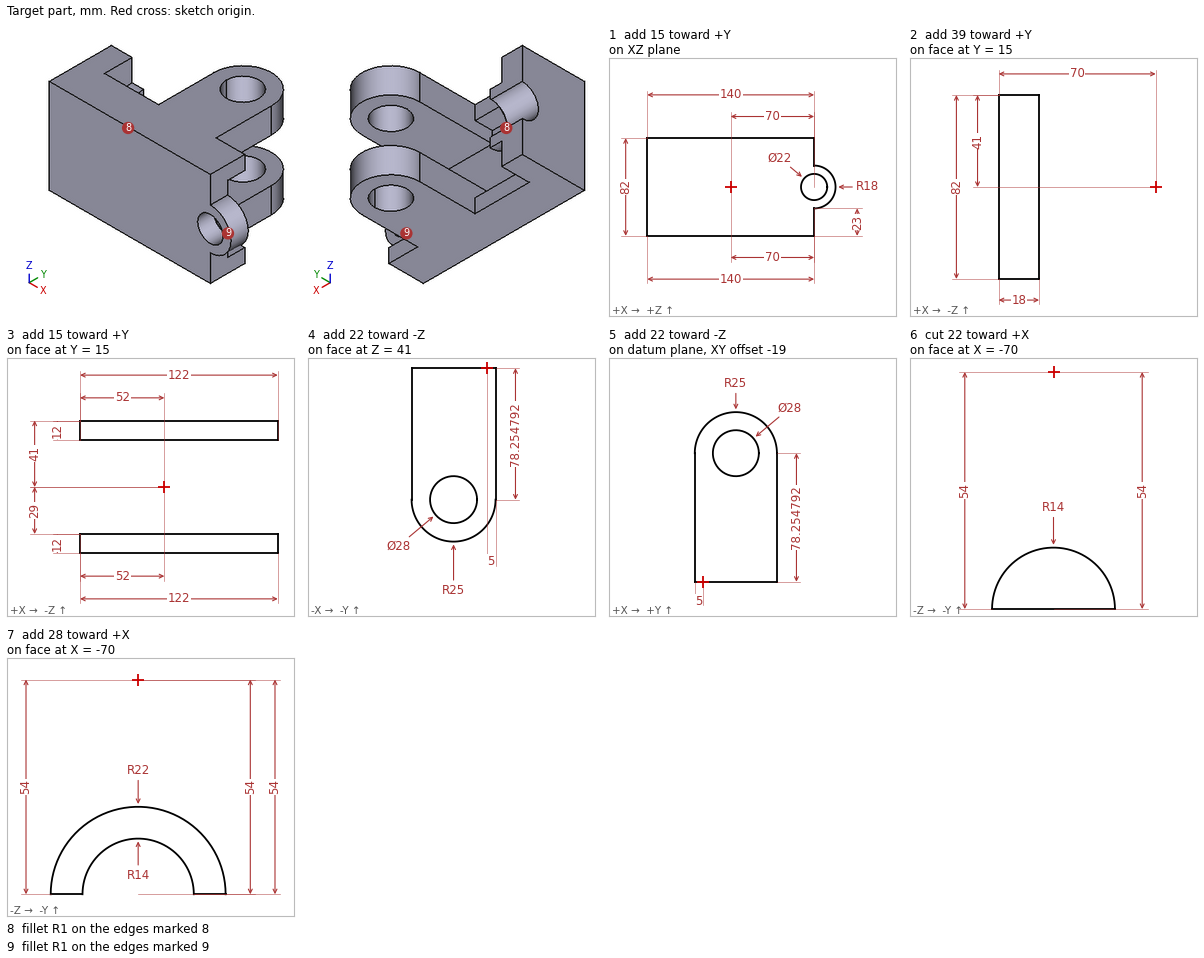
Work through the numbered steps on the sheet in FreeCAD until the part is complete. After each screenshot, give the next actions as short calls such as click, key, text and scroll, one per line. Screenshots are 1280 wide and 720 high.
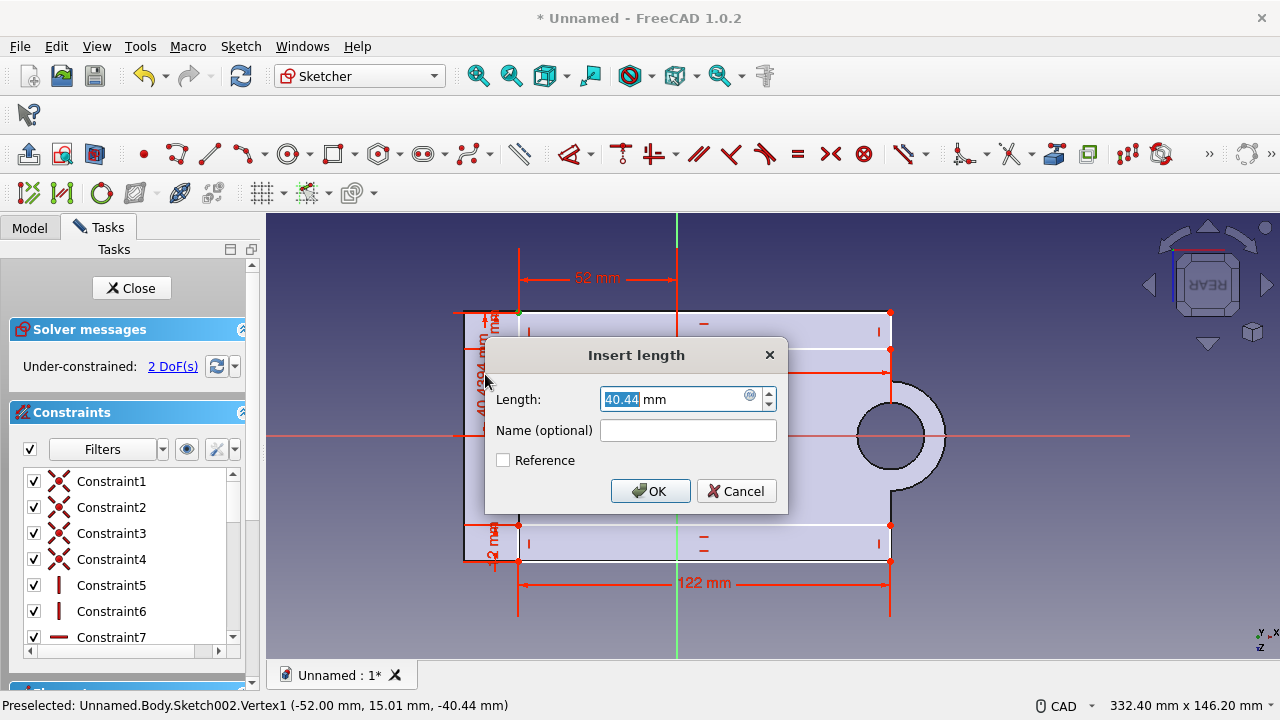
text(41)
key(Return)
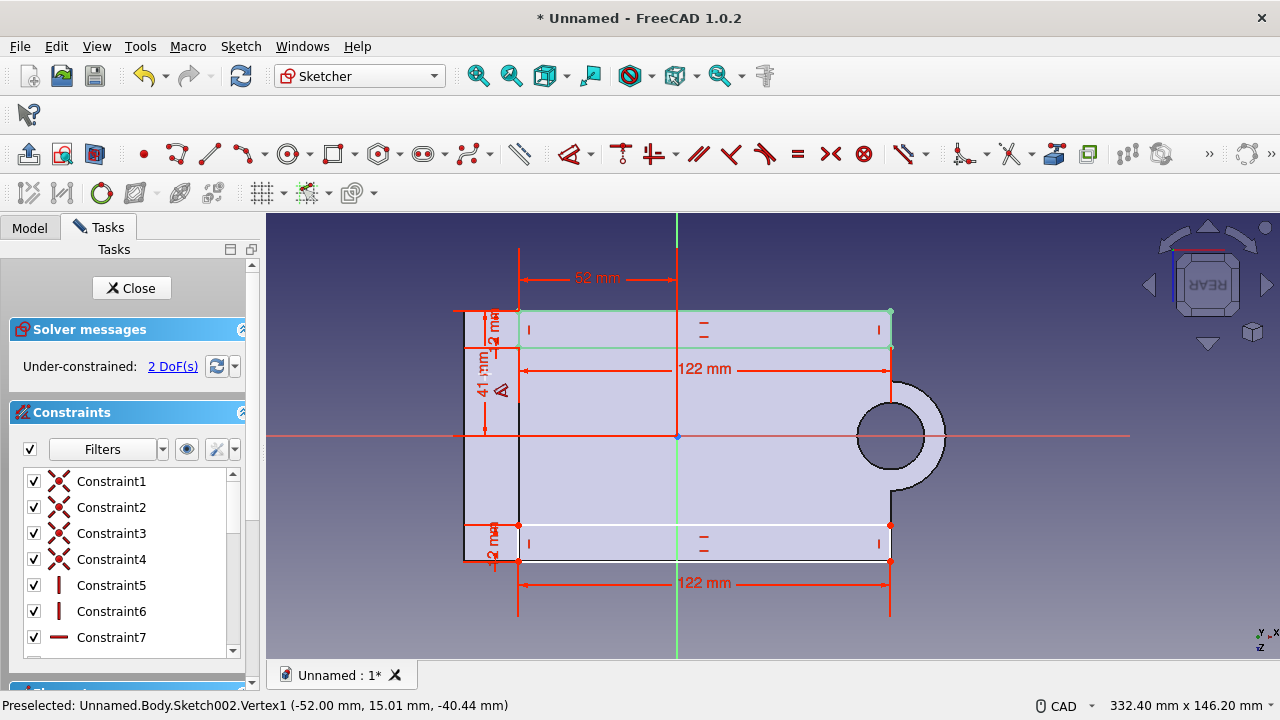
click(518, 525)
click(598, 402)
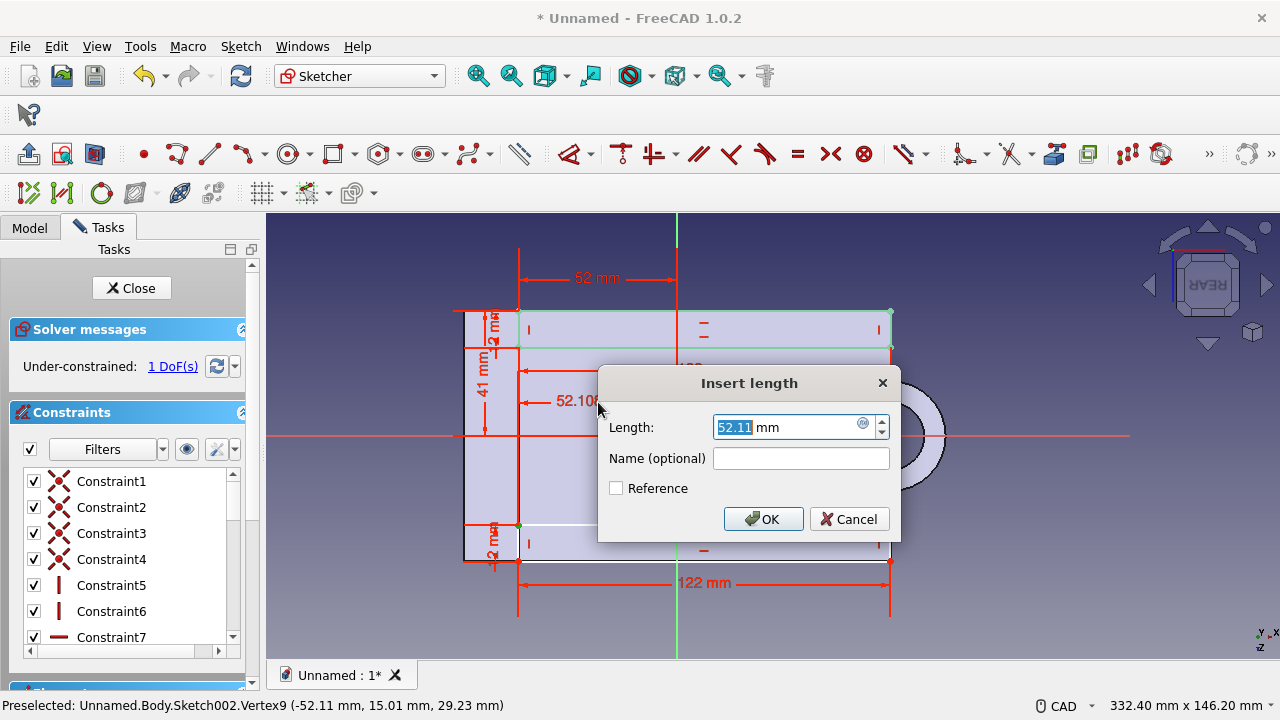
text(52)
key(Return)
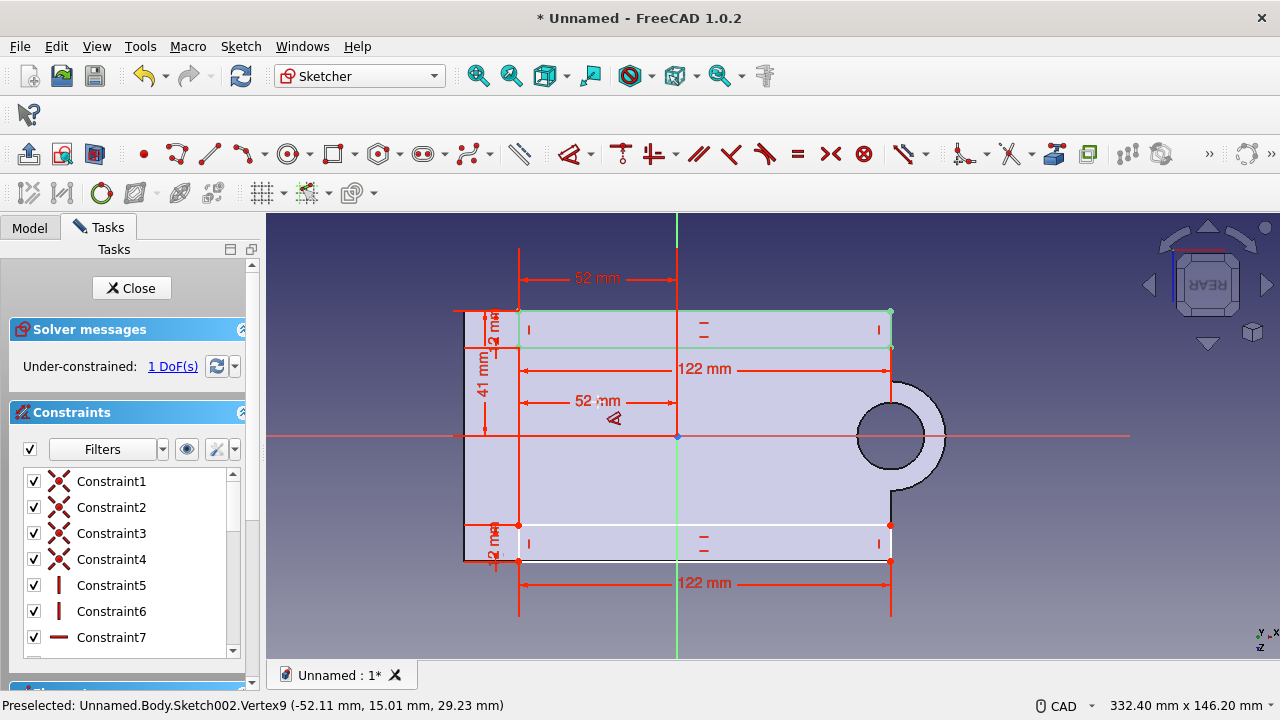
click(519, 525)
click(485, 481)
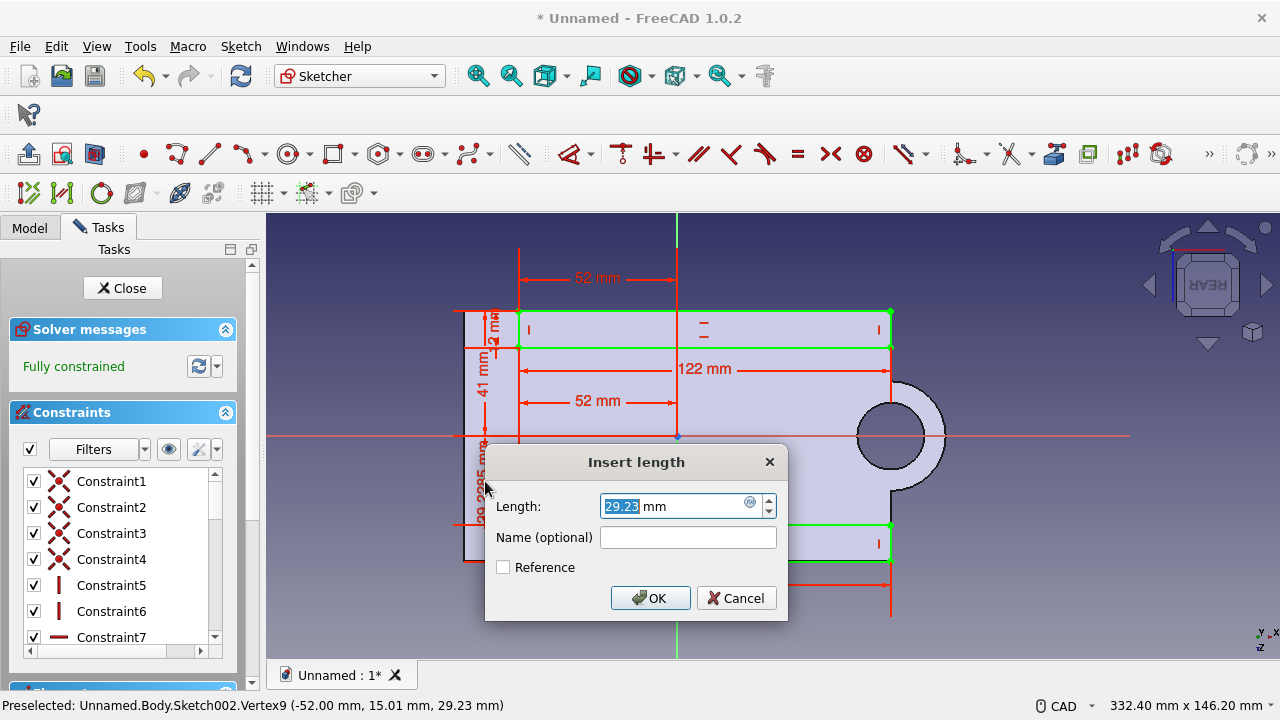
text(29)
key(Return)
key(Escape)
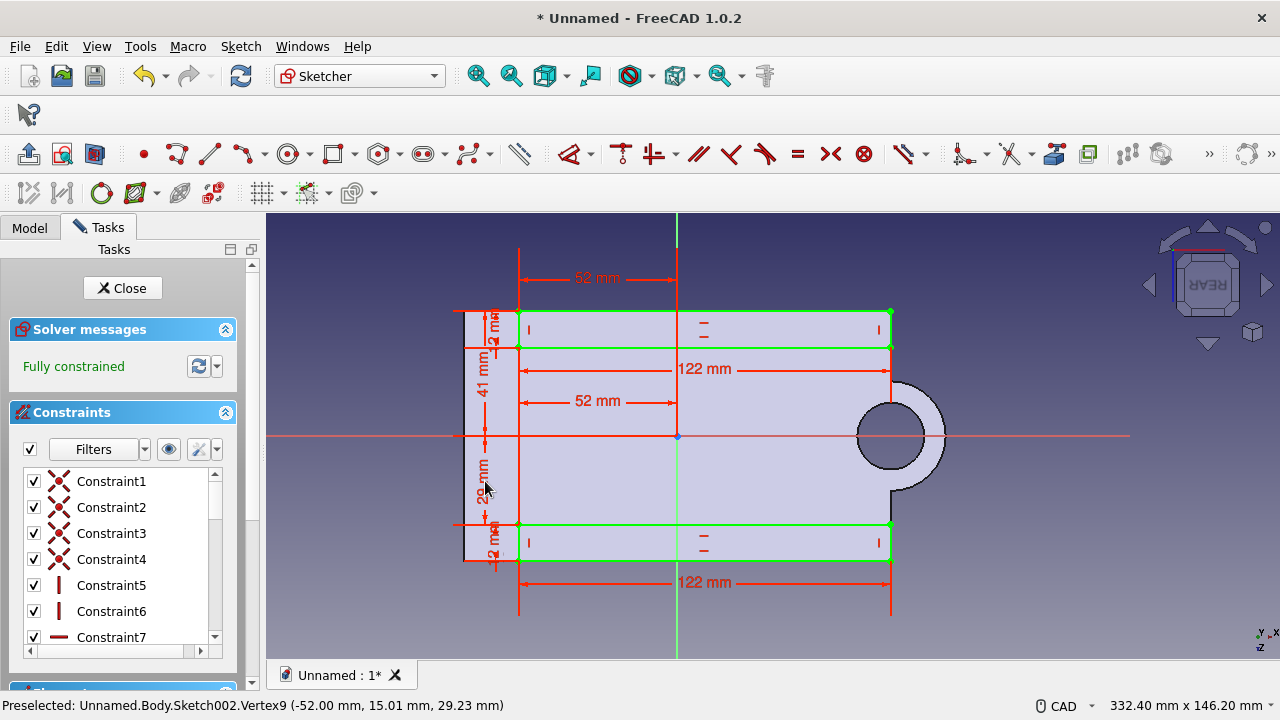
click(123, 288)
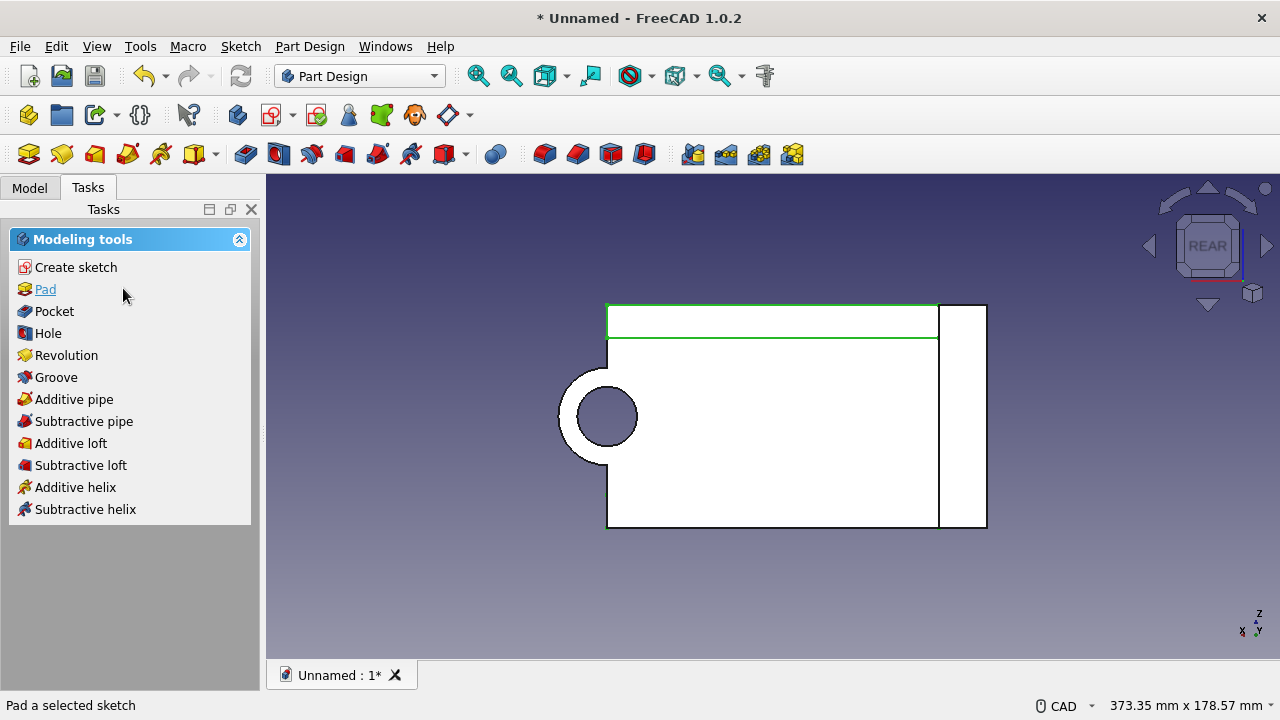
click(29, 154)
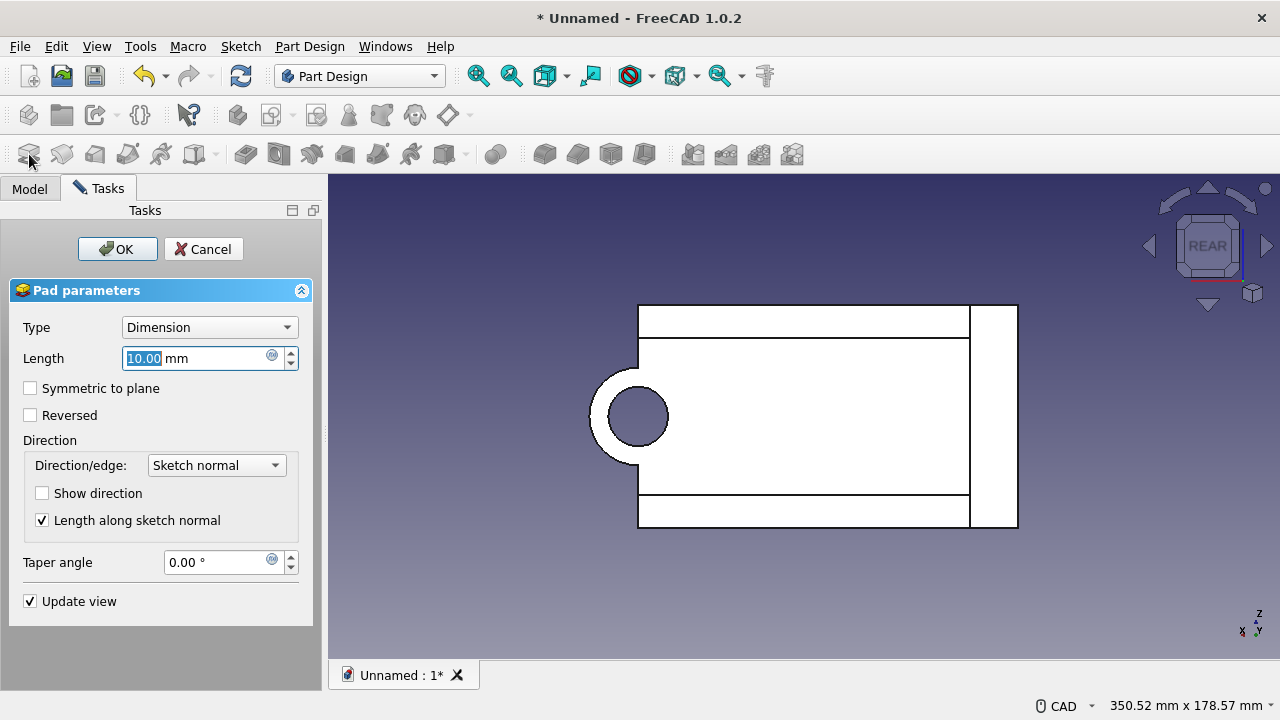
text(15)
key(Tab)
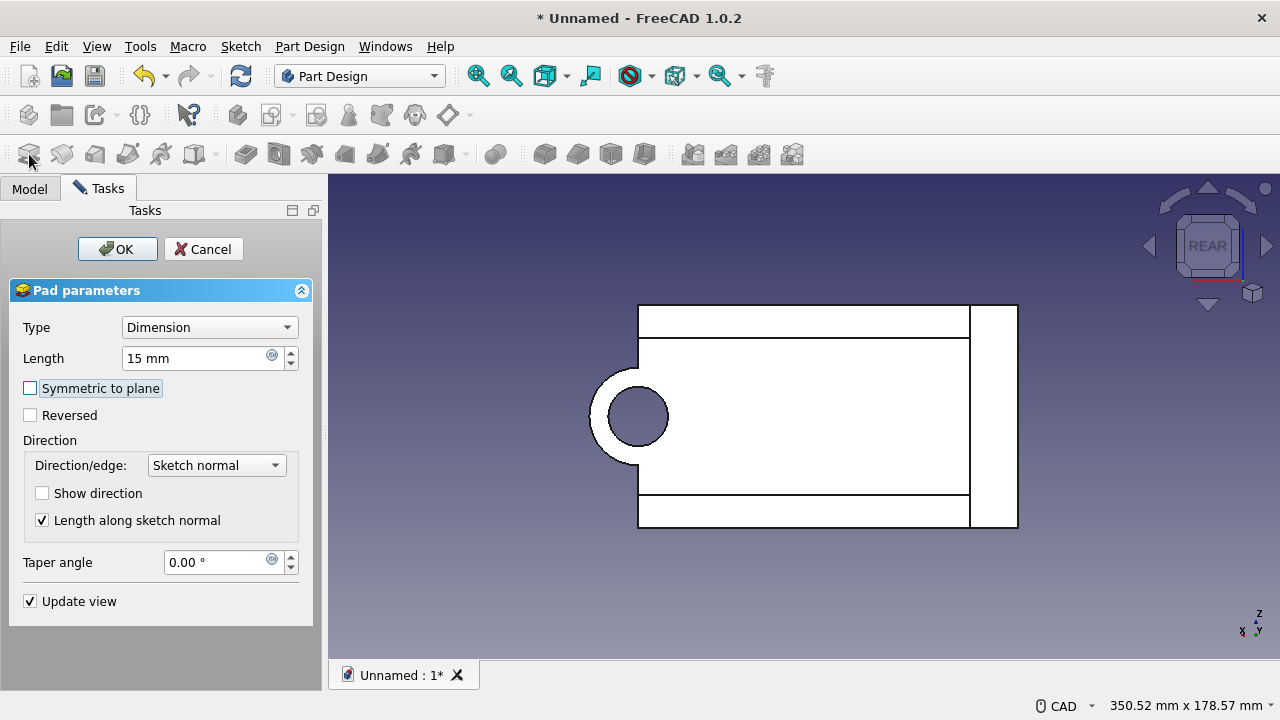
click(118, 249)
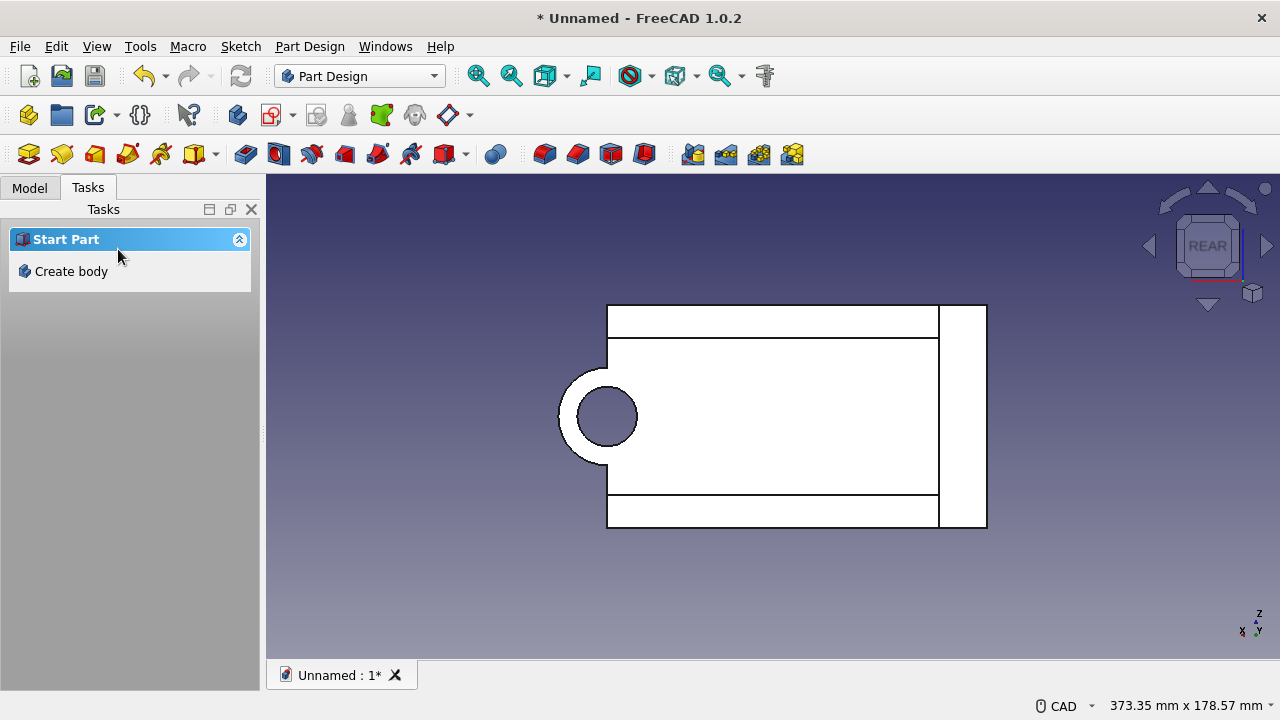
key(0)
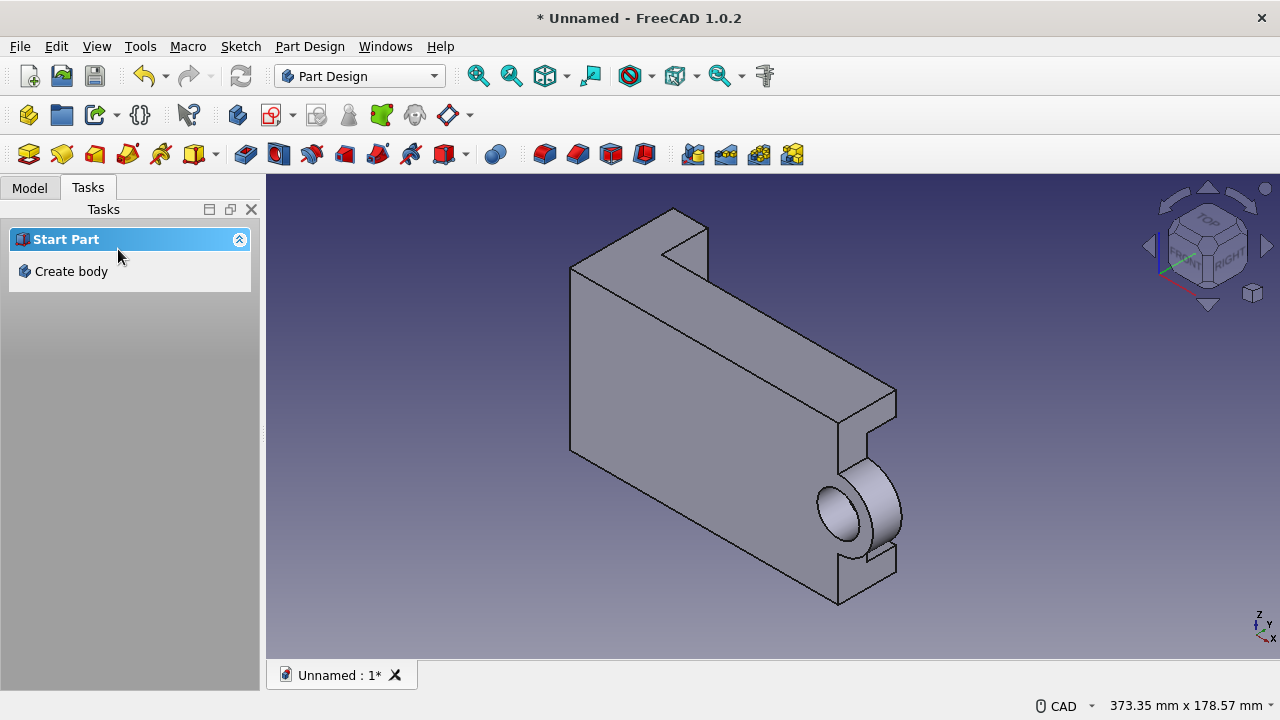
click(803, 376)